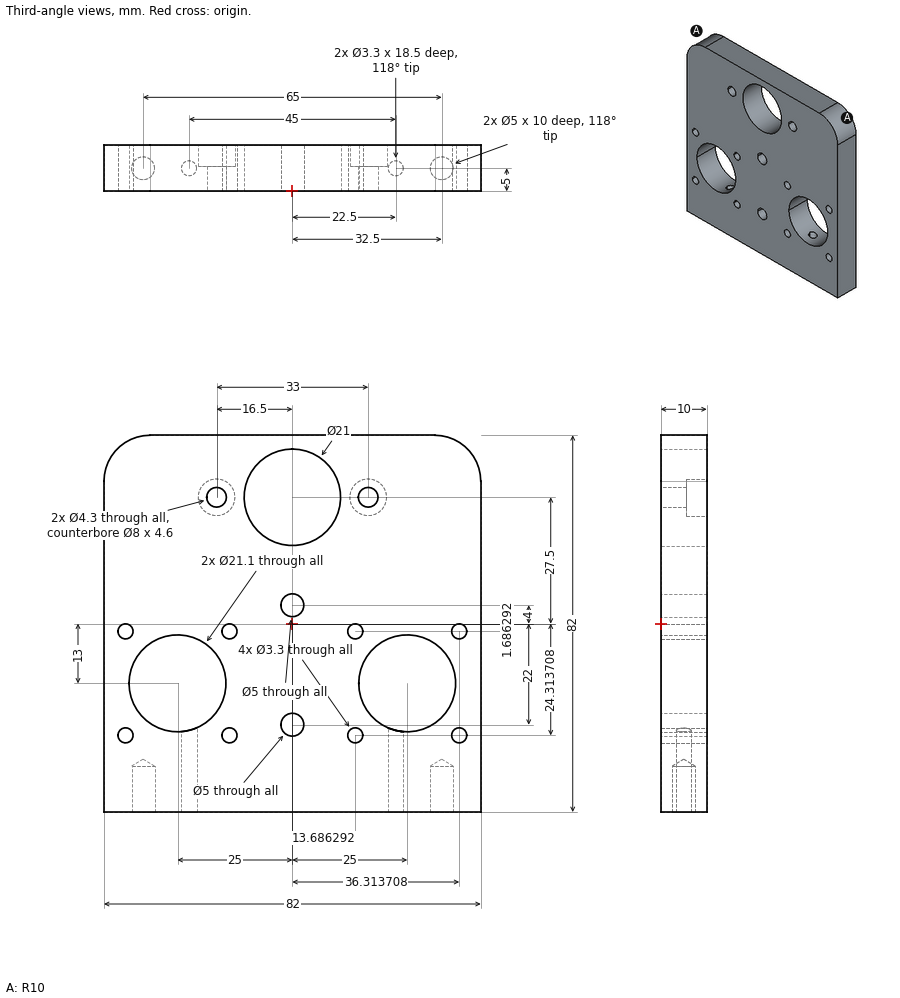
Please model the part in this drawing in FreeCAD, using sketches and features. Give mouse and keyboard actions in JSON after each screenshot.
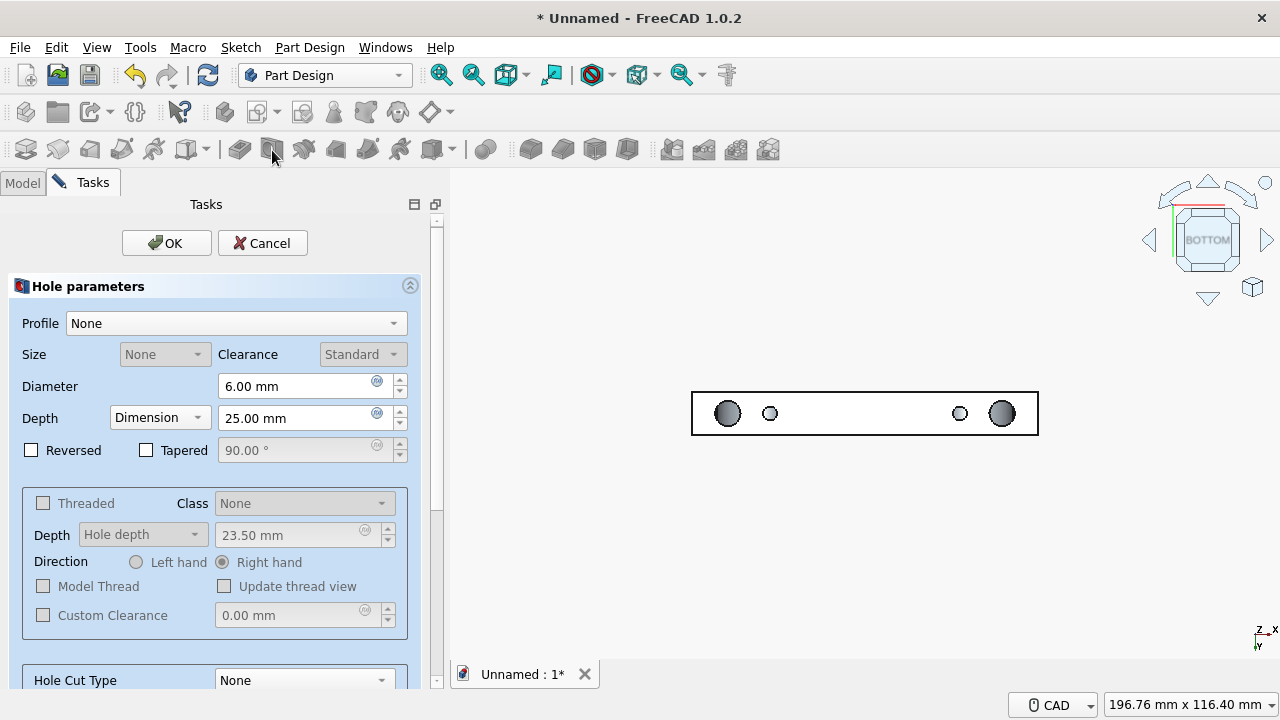
{"action": "triple_click", "coordinate": [305, 386]}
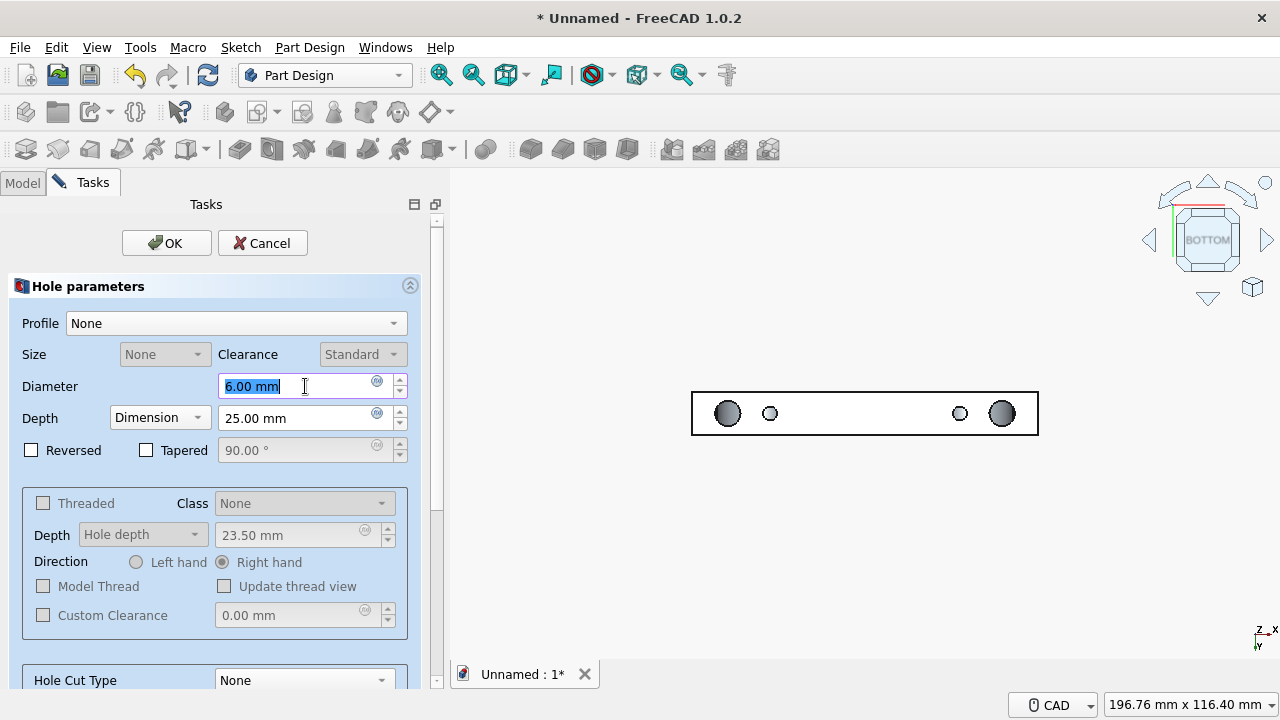
{"action": "type", "text": "5"}
{"action": "key", "text": "Tab"}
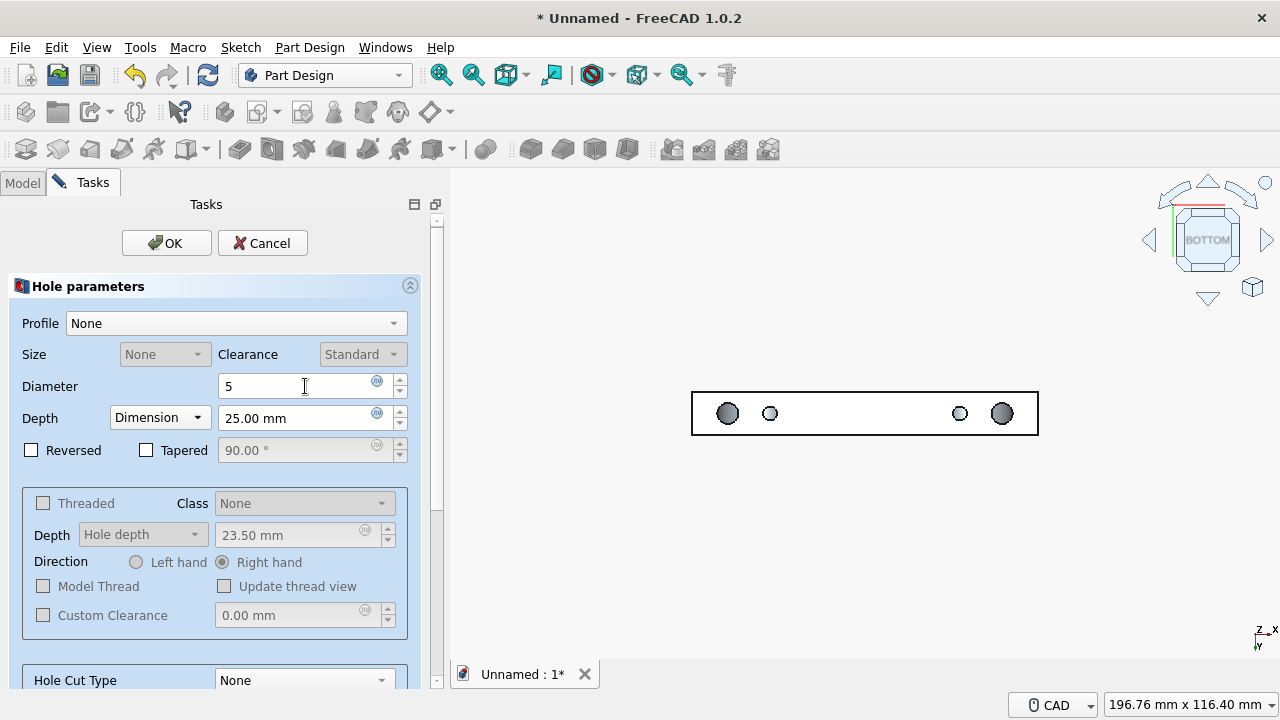
{"action": "triple_click", "coordinate": [305, 418]}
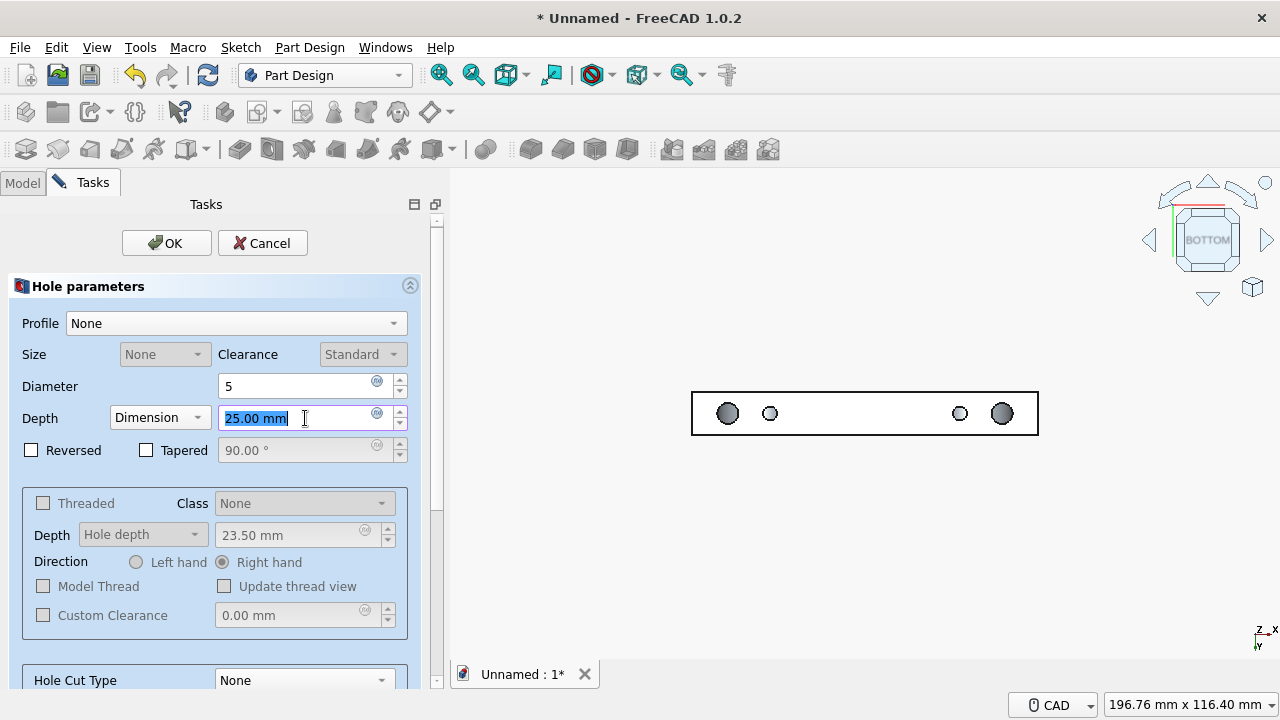
{"action": "type", "text": "10"}
{"action": "key", "text": "Tab"}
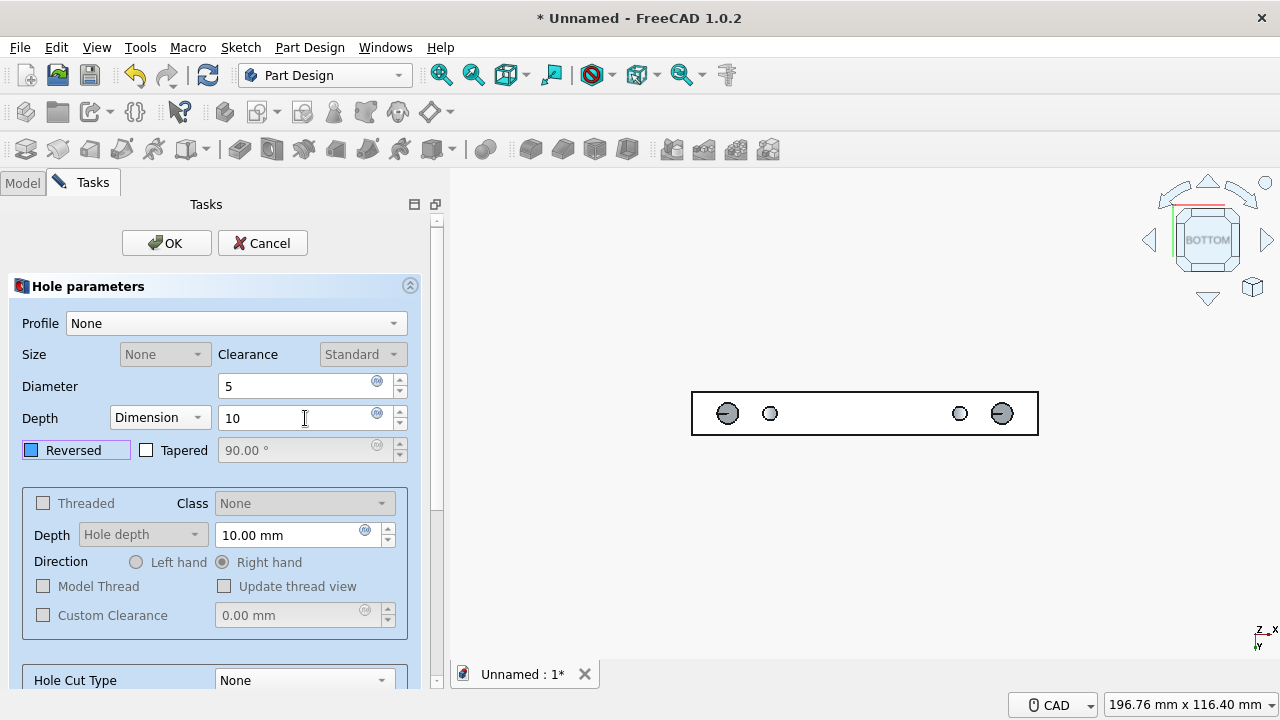
{"action": "left_click", "coordinate": [167, 243]}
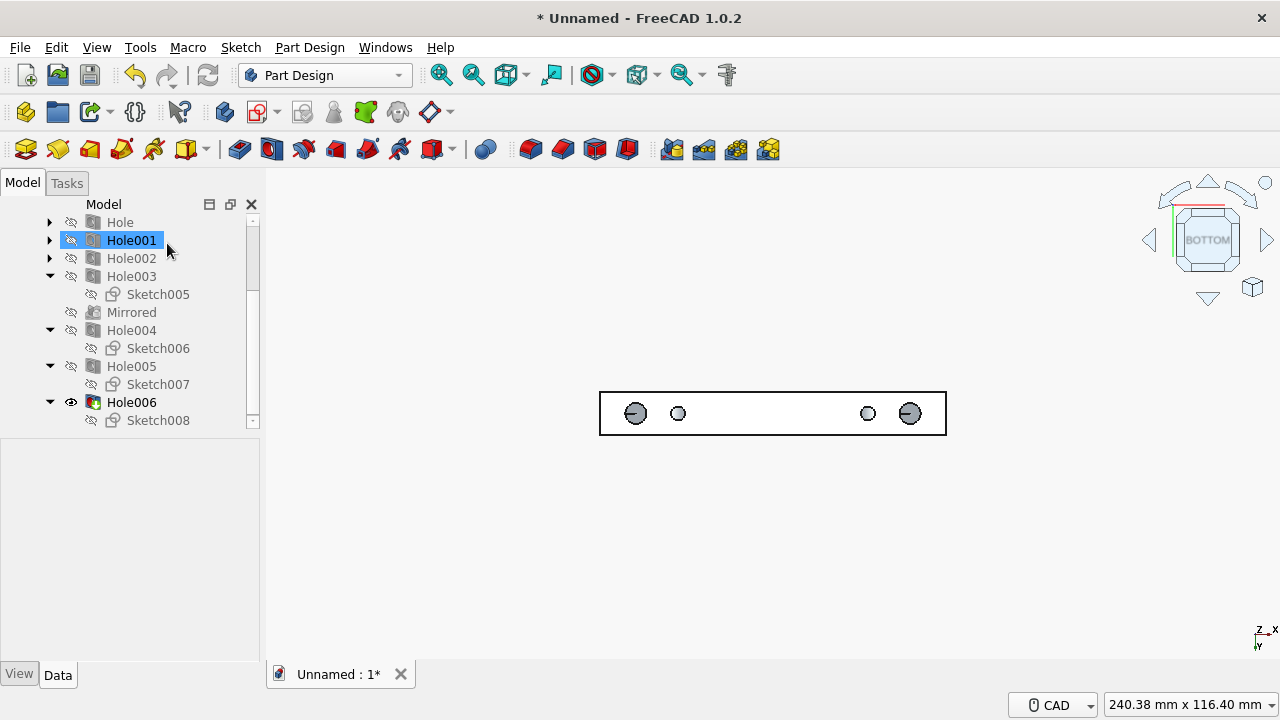
{"action": "key", "text": "0"}